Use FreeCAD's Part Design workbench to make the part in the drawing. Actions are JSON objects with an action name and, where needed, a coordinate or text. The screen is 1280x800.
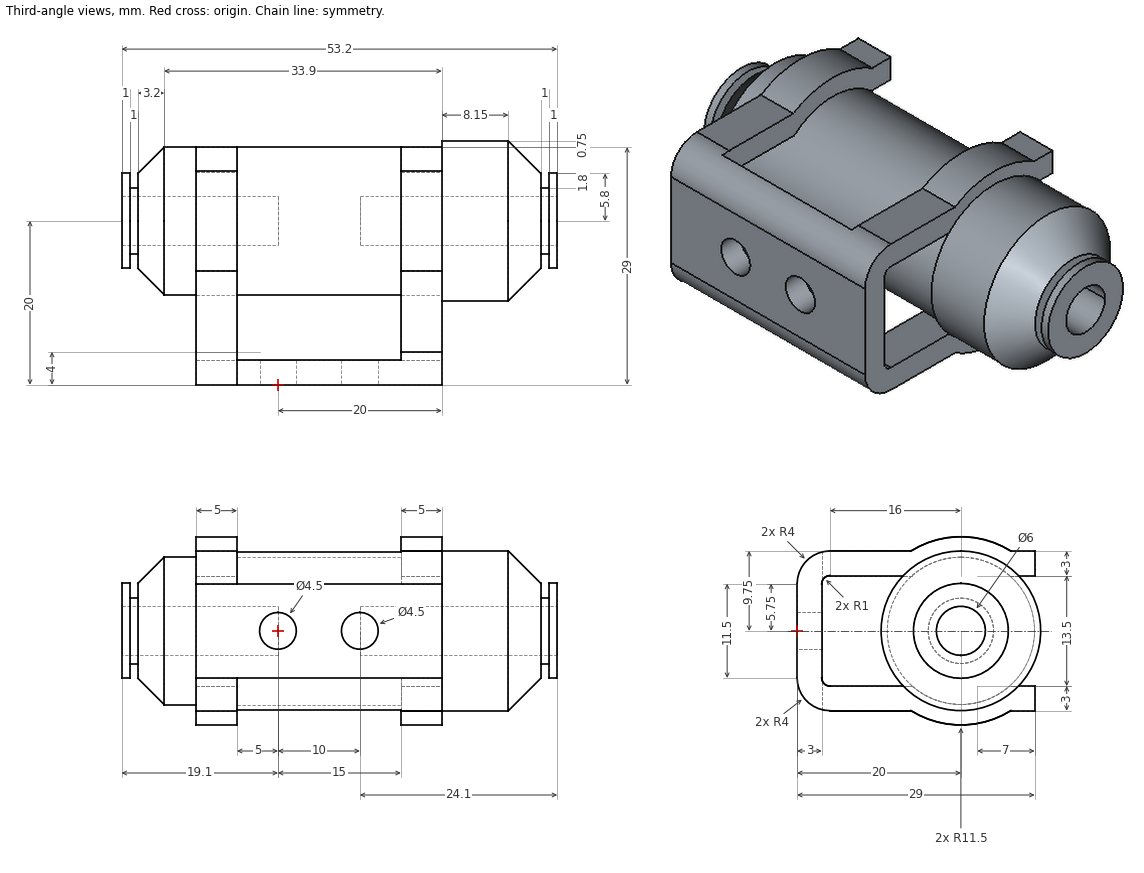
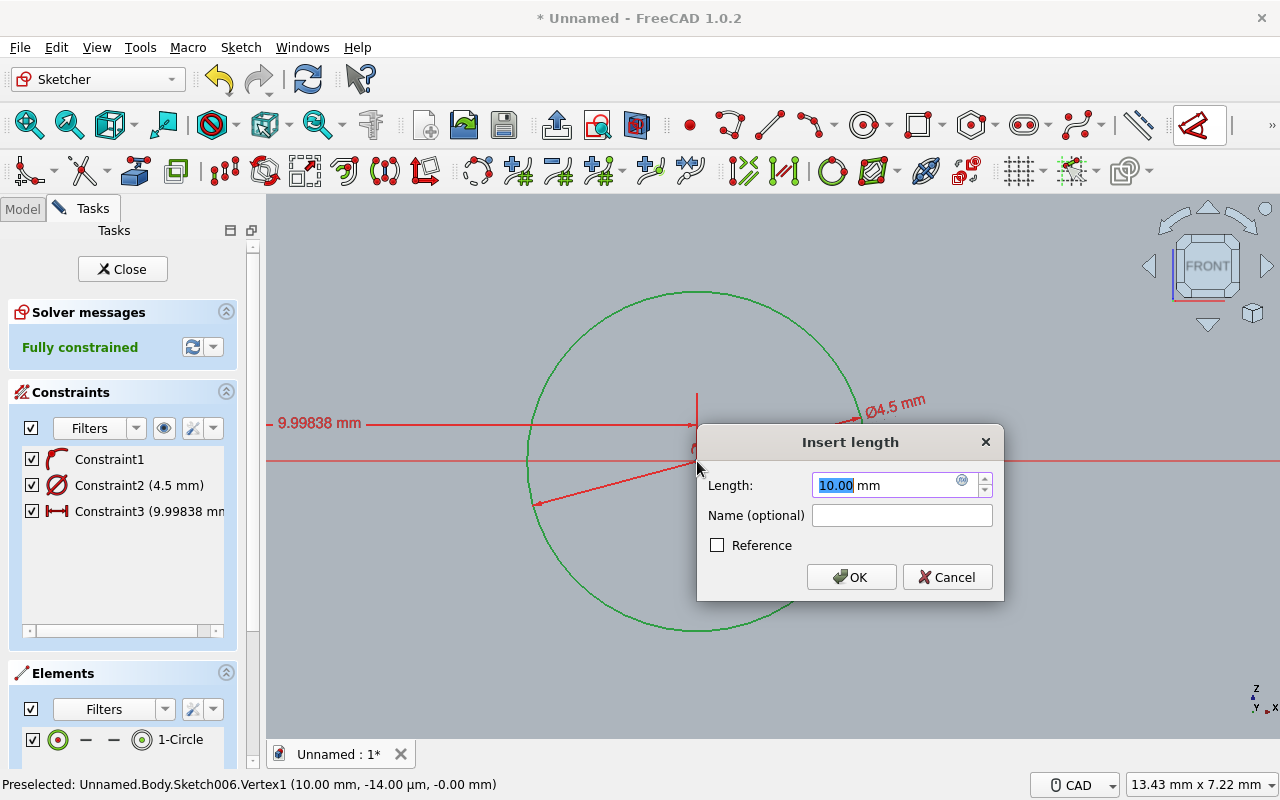
{"action": "type", "text": "10"}
{"action": "key", "text": "Return"}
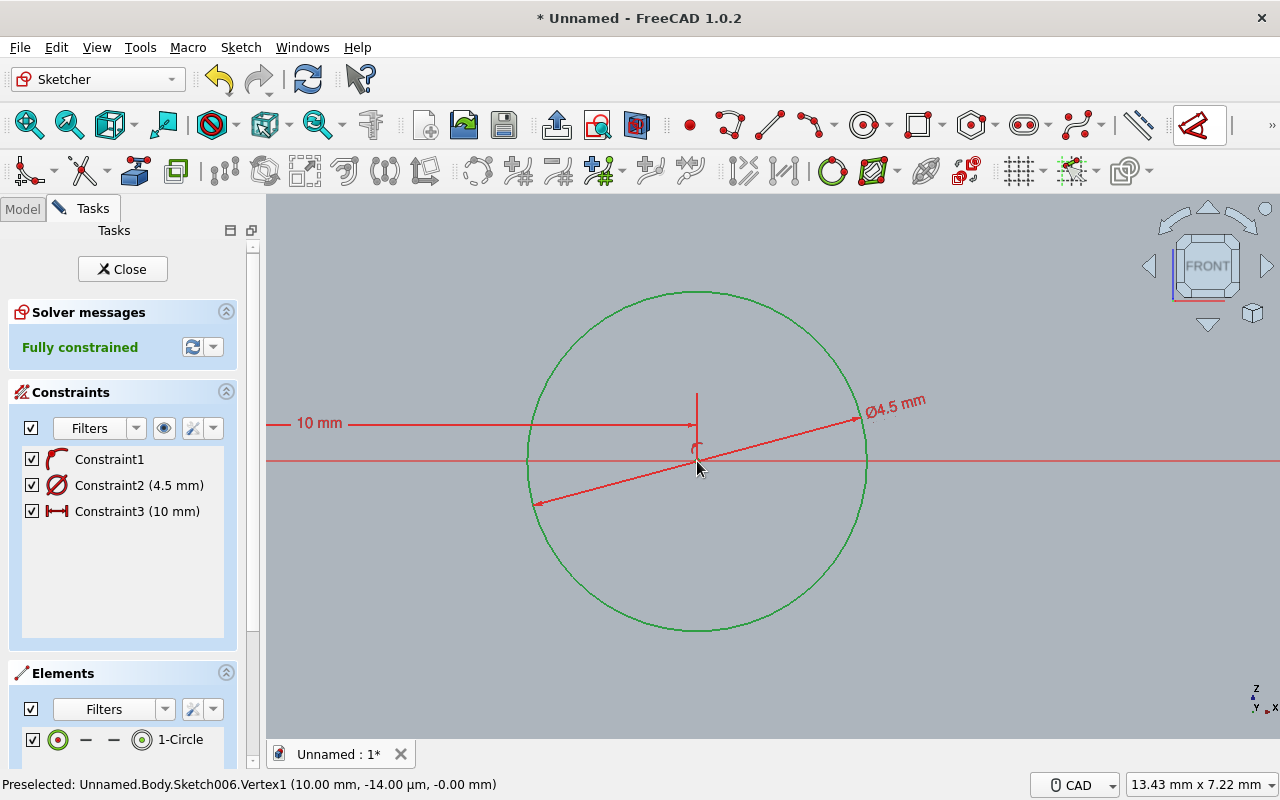
{"action": "left_click", "coordinate": [123, 269]}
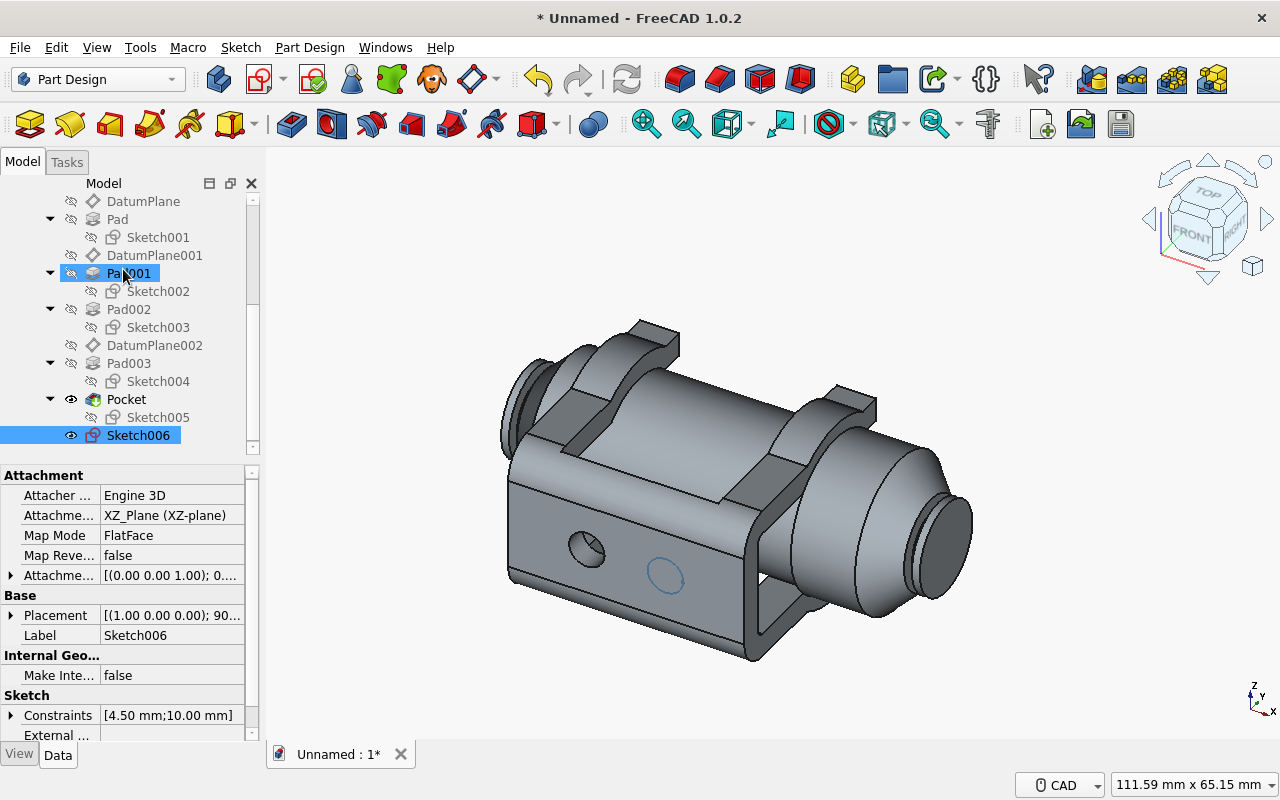
{"action": "left_click", "coordinate": [292, 124]}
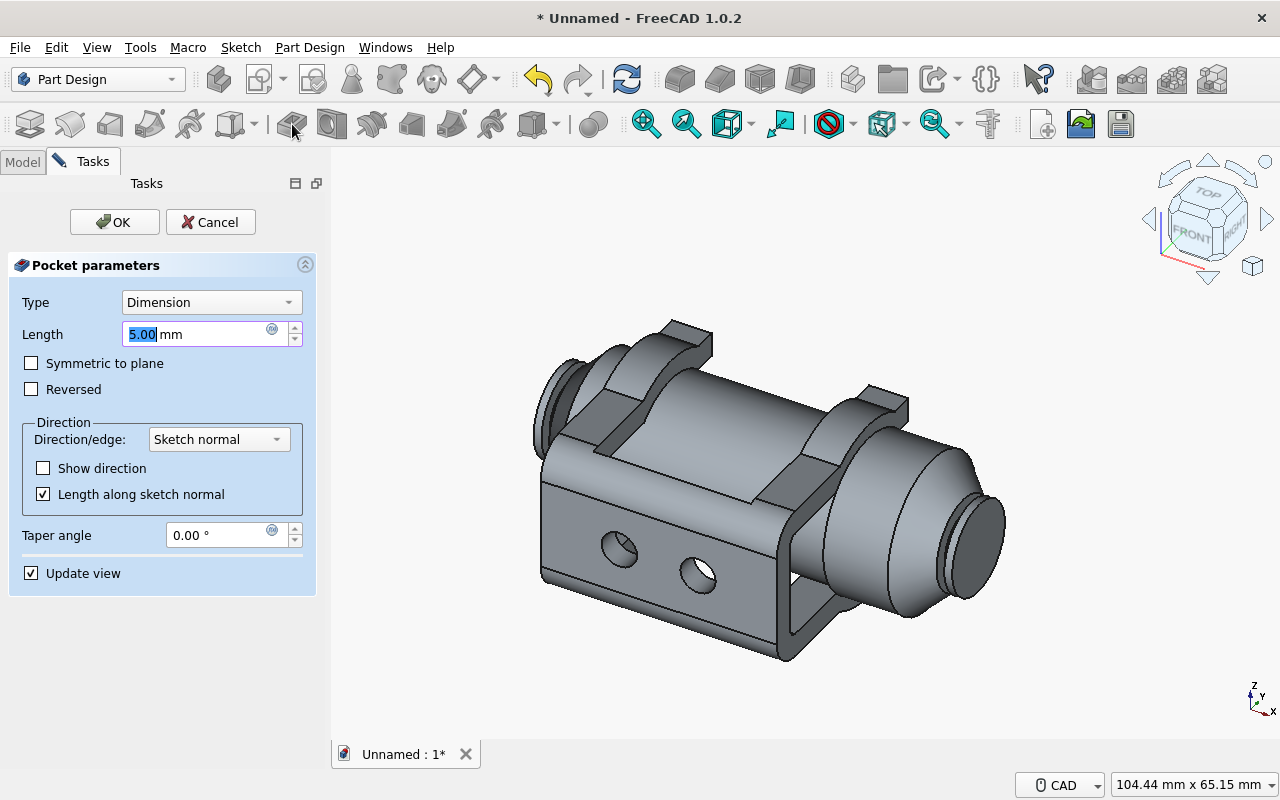
{"action": "type", "text": "4"}
{"action": "key", "text": "Tab"}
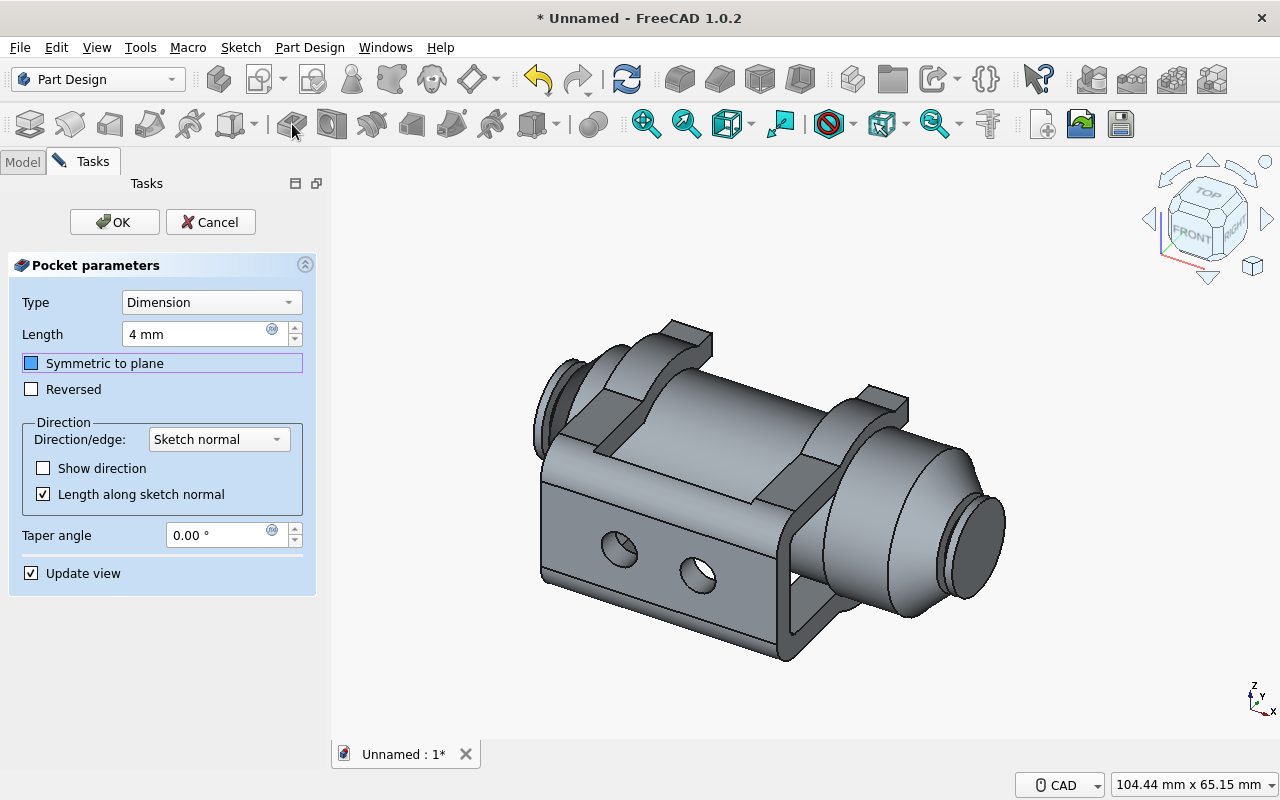
{"action": "left_click", "coordinate": [115, 222]}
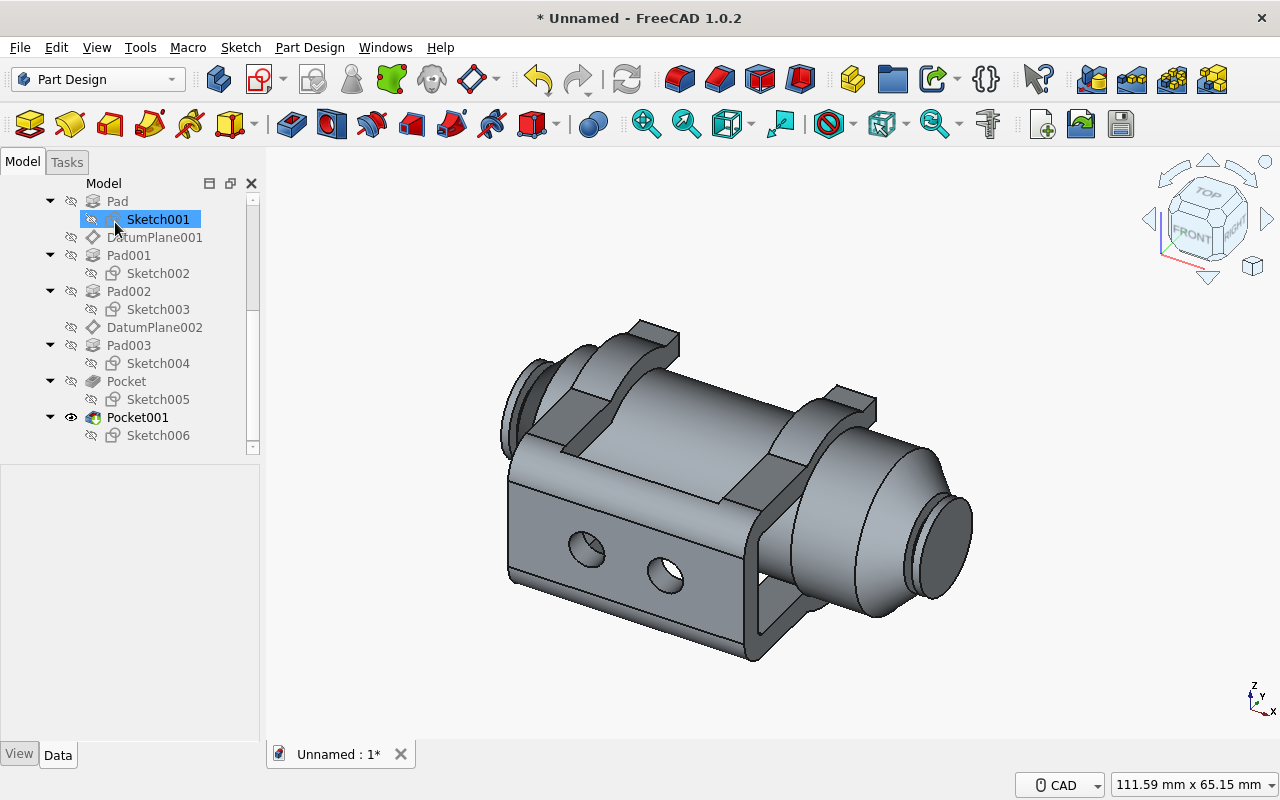
{"action": "left_click", "coordinate": [946, 547]}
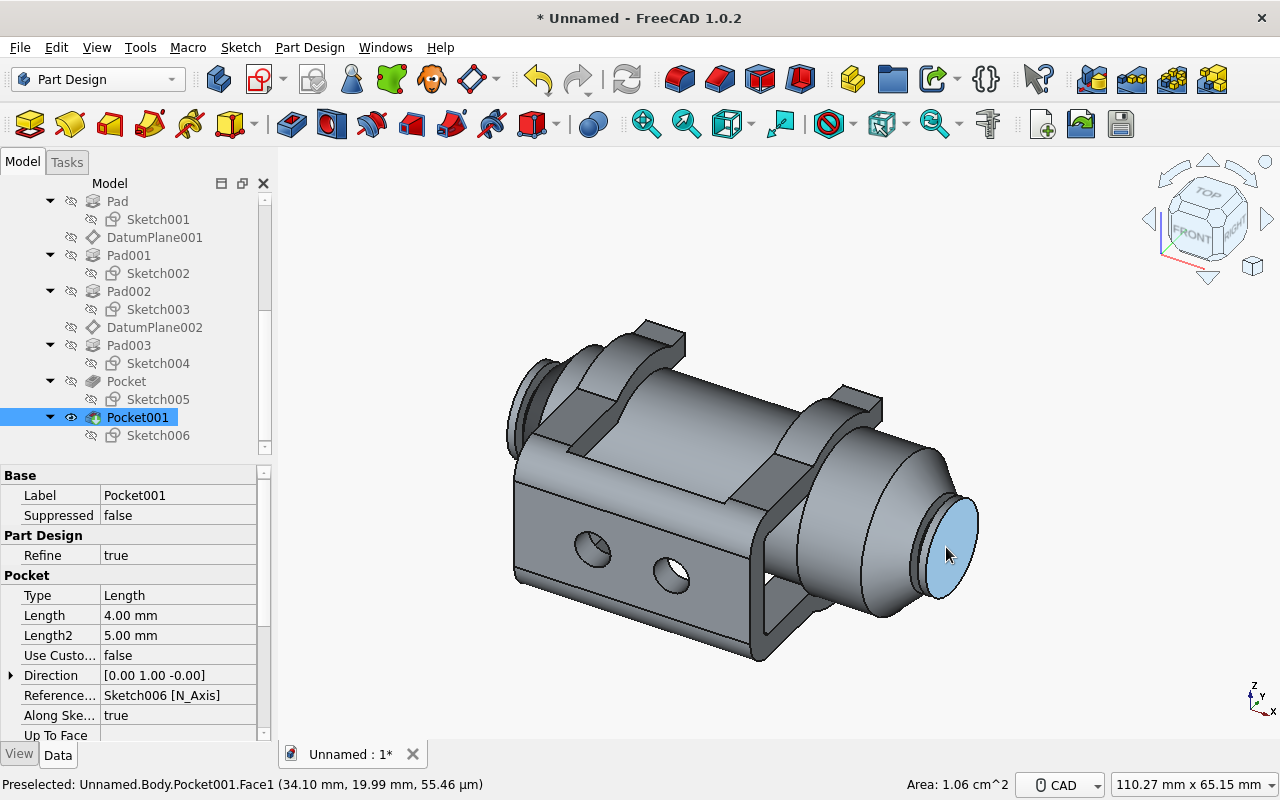
{"action": "left_click", "coordinate": [260, 80]}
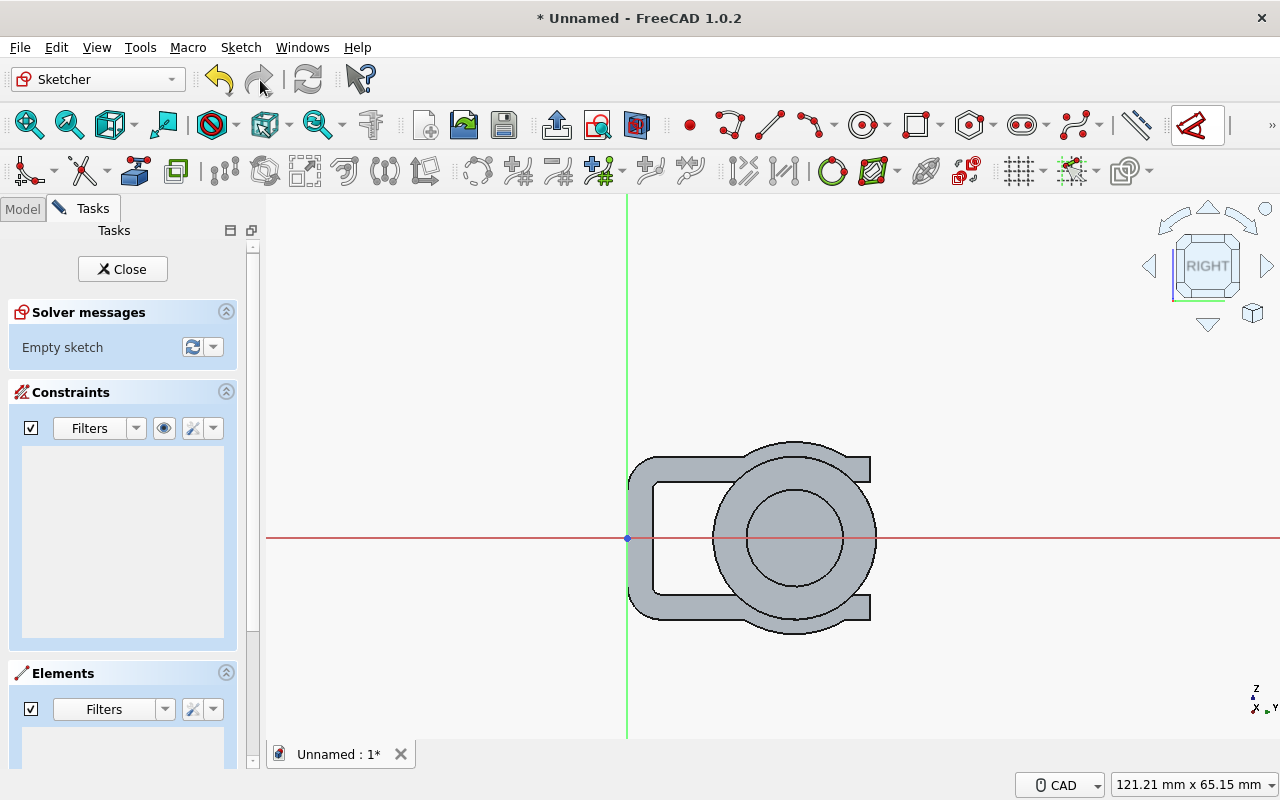
{"action": "scroll", "coordinate": [809, 549], "scroll_direction": "up", "scroll_amount": 10}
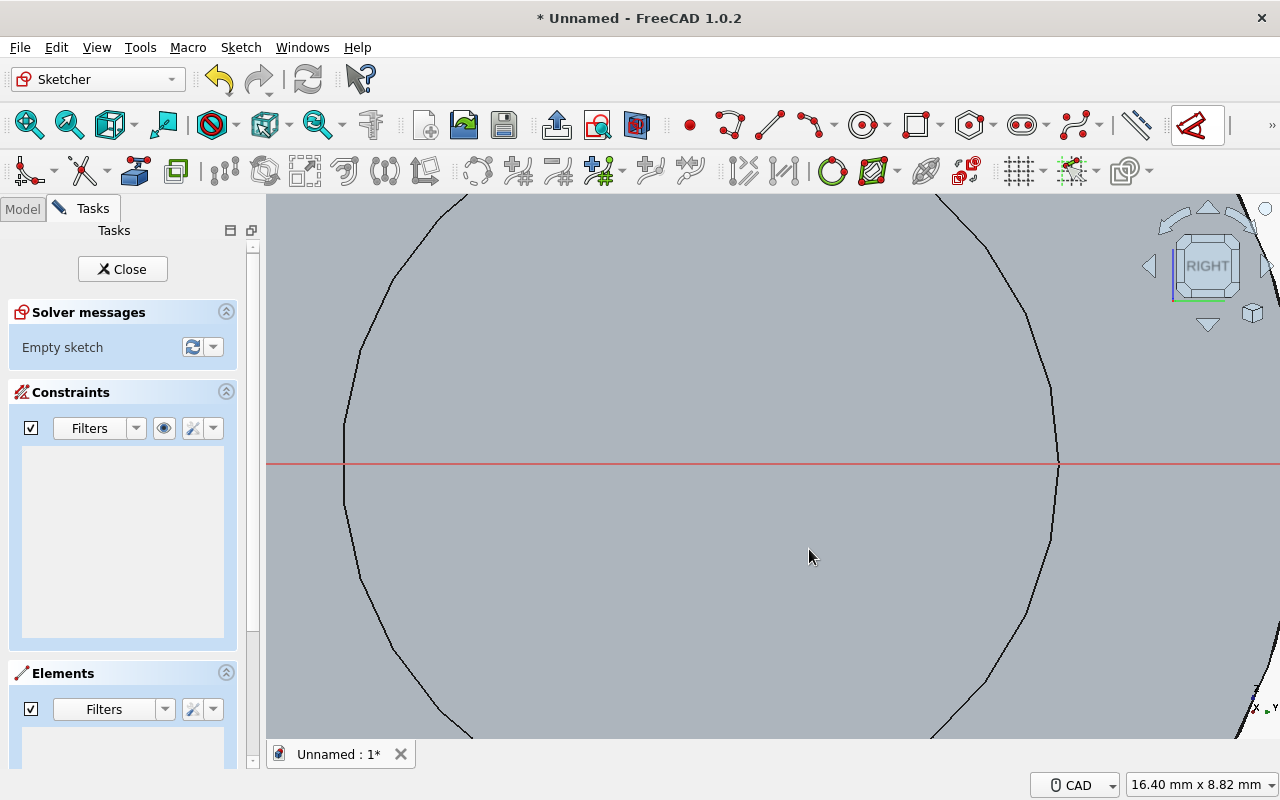
{"action": "left_click", "coordinate": [864, 126]}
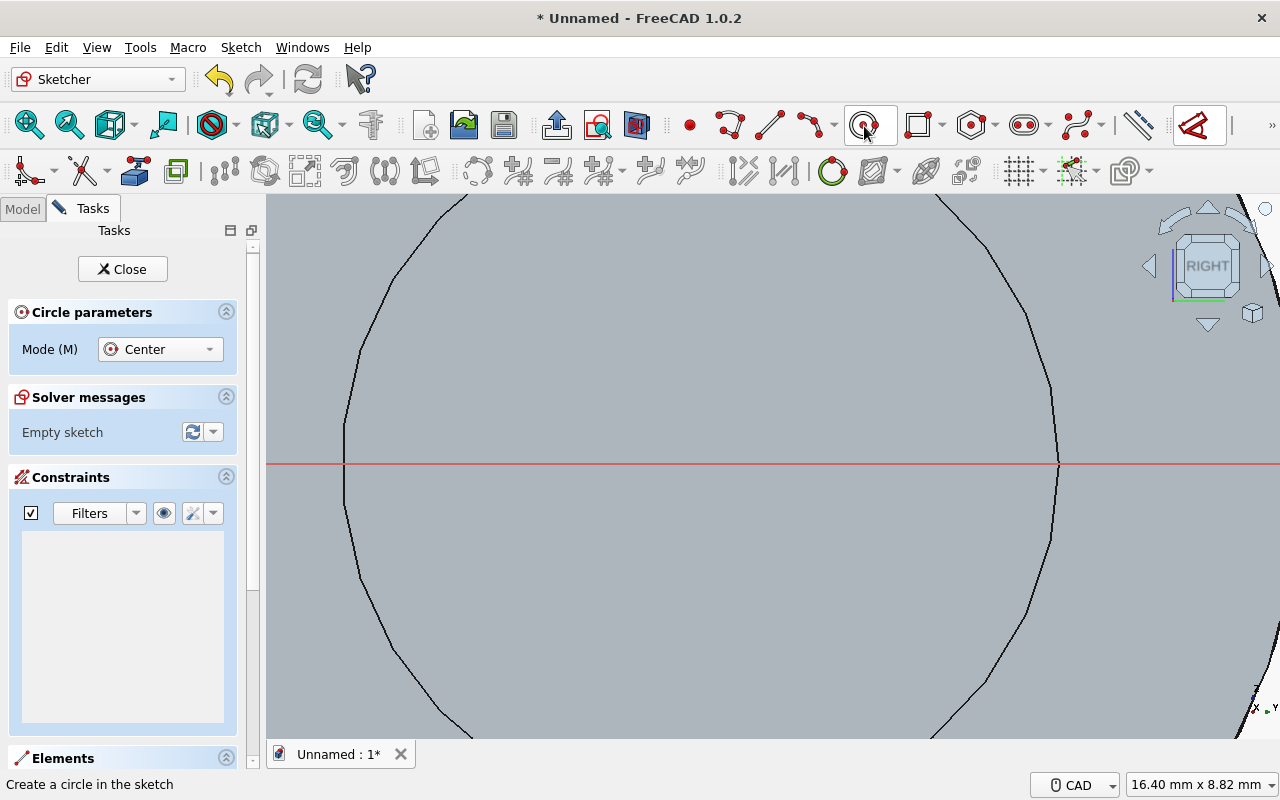
{"action": "left_click", "coordinate": [700, 464]}
{"action": "left_click", "coordinate": [831, 333]}
{"action": "key", "text": "Escape"}